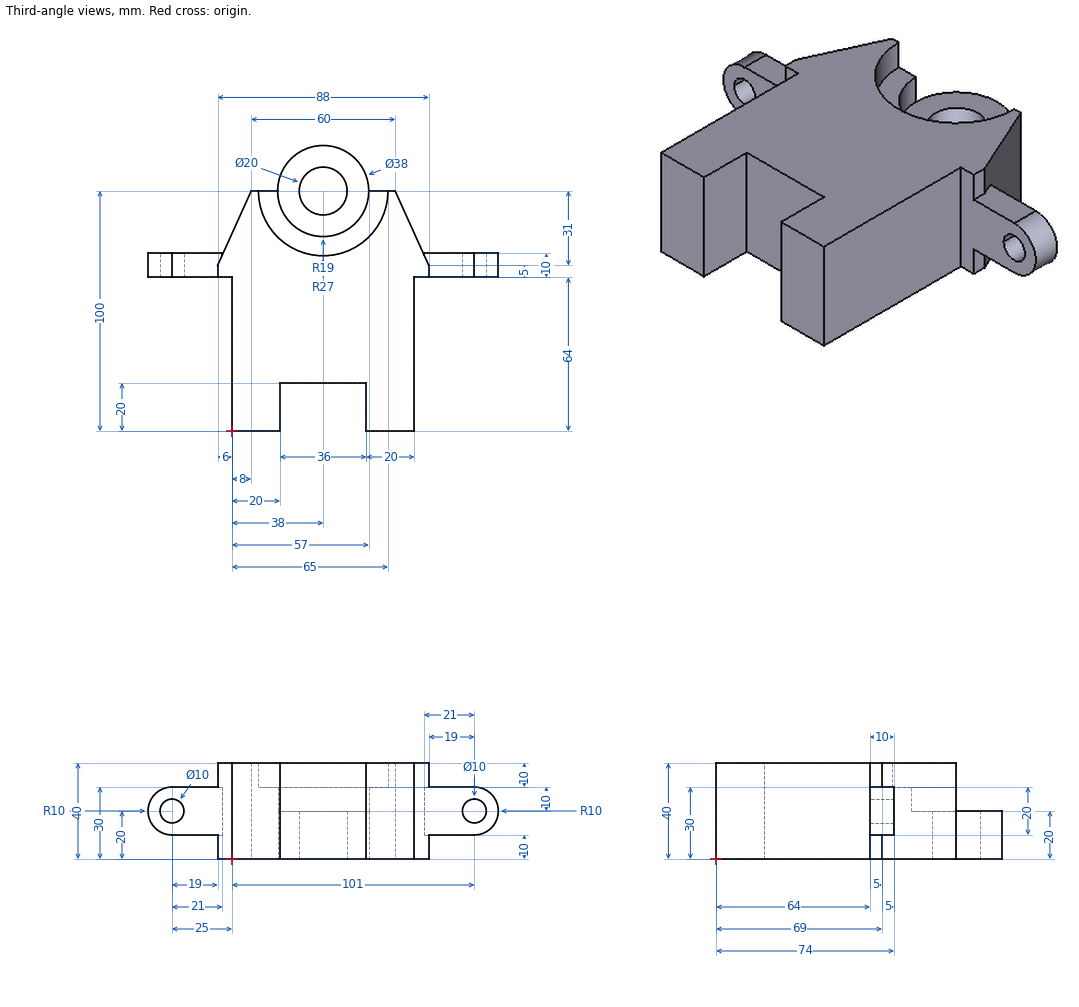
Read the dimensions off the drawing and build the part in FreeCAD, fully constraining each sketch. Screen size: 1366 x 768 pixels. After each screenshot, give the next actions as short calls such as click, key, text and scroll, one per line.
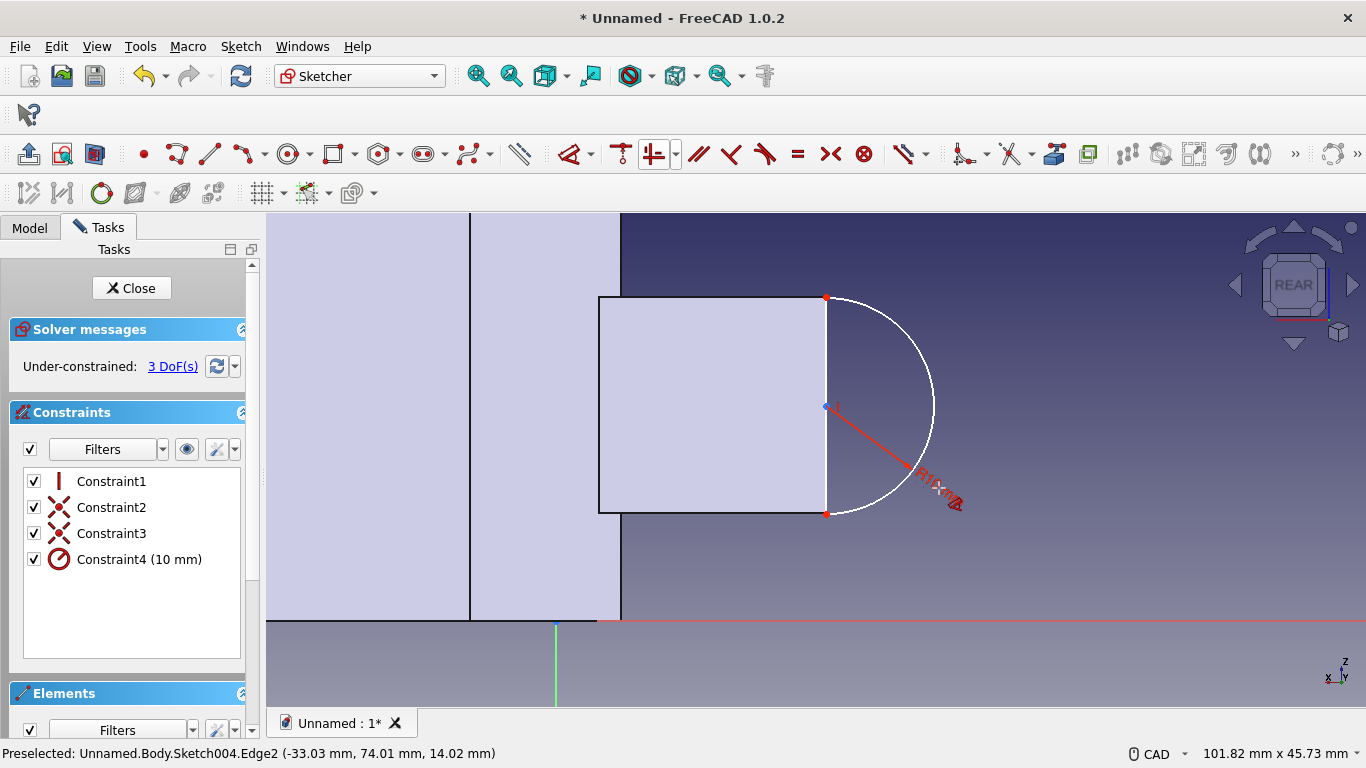
click(826, 298)
click(691, 655)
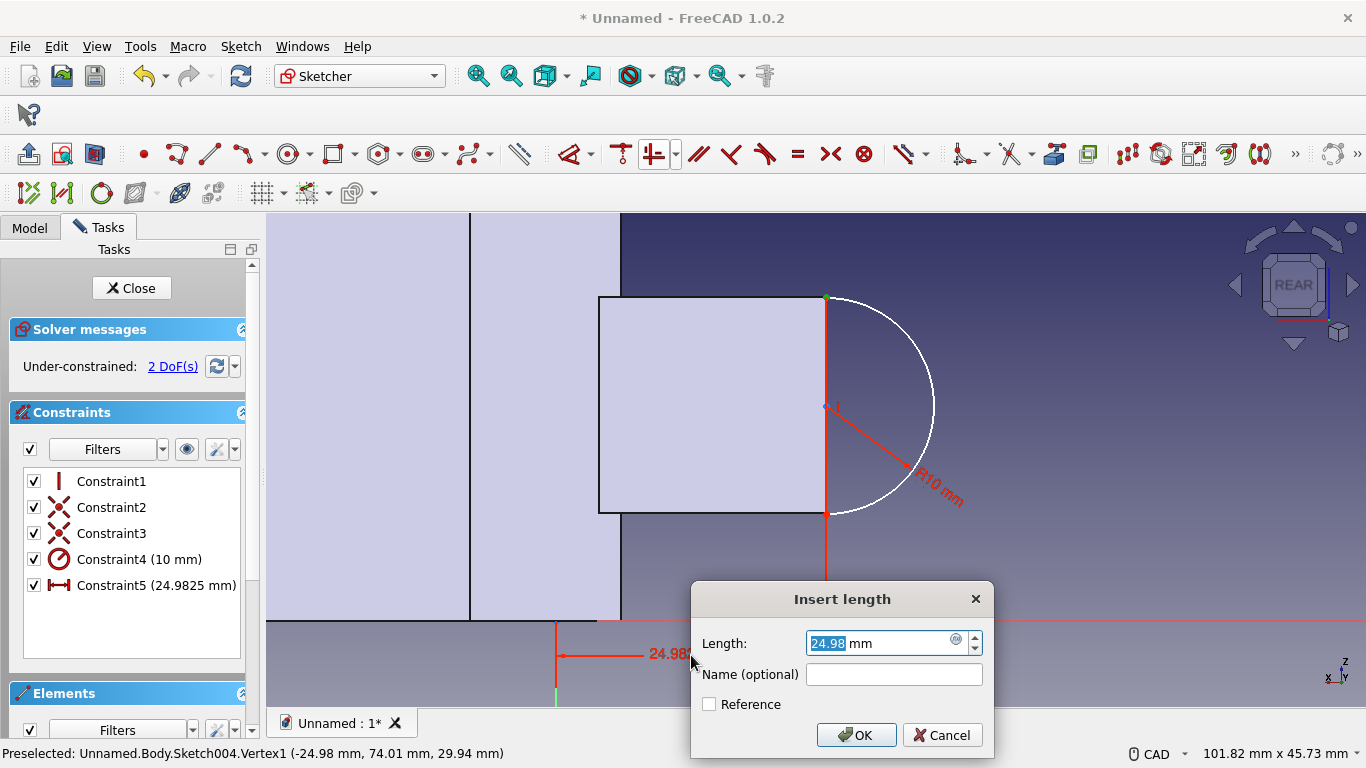
text(25)
key(Return)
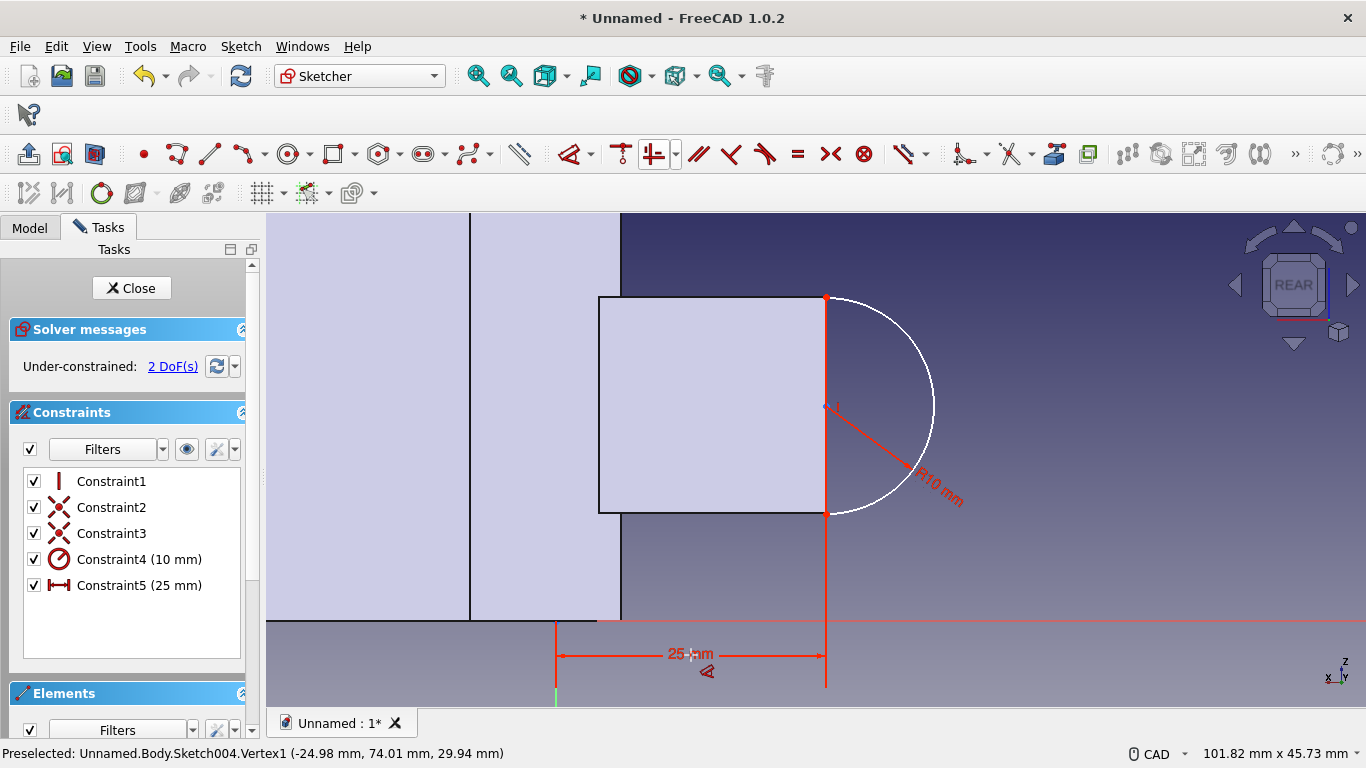
click(826, 298)
click(522, 460)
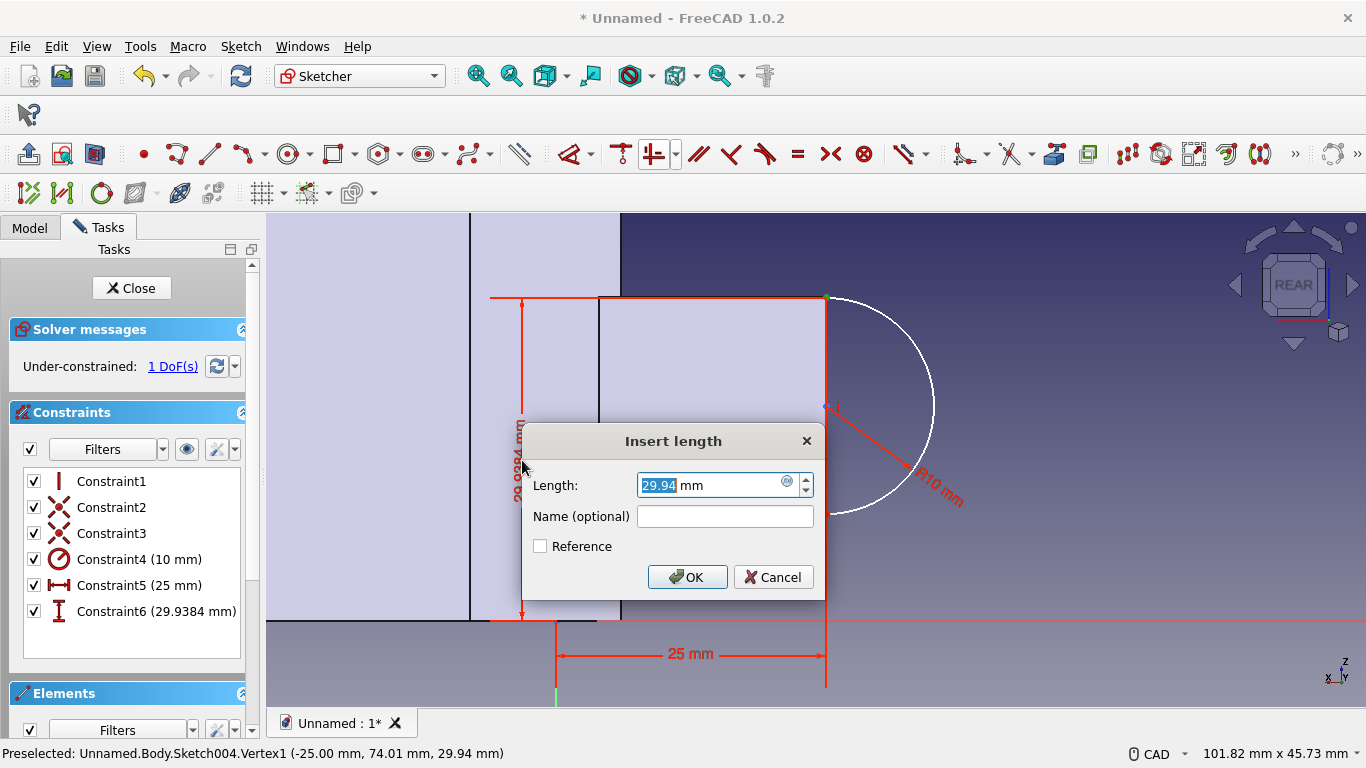
text(30)
key(Return)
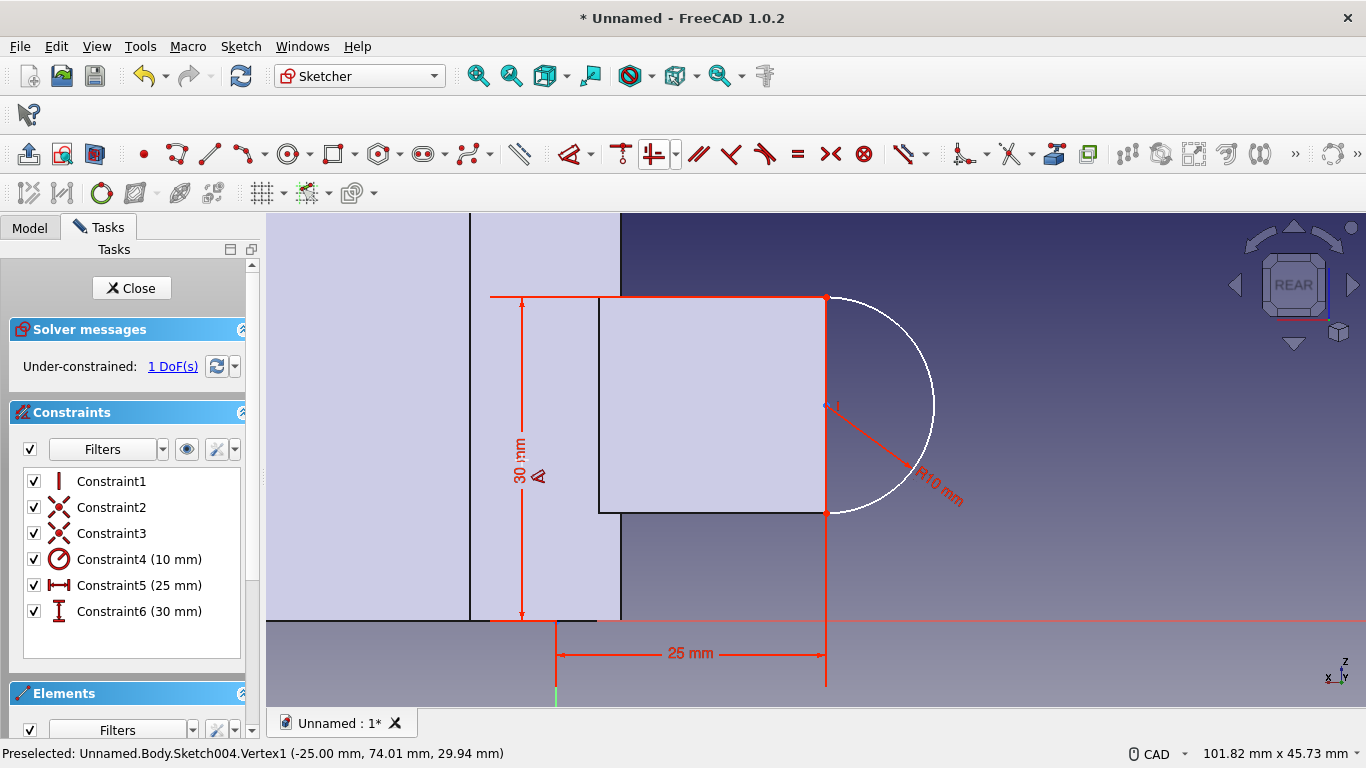
click(826, 405)
click(597, 655)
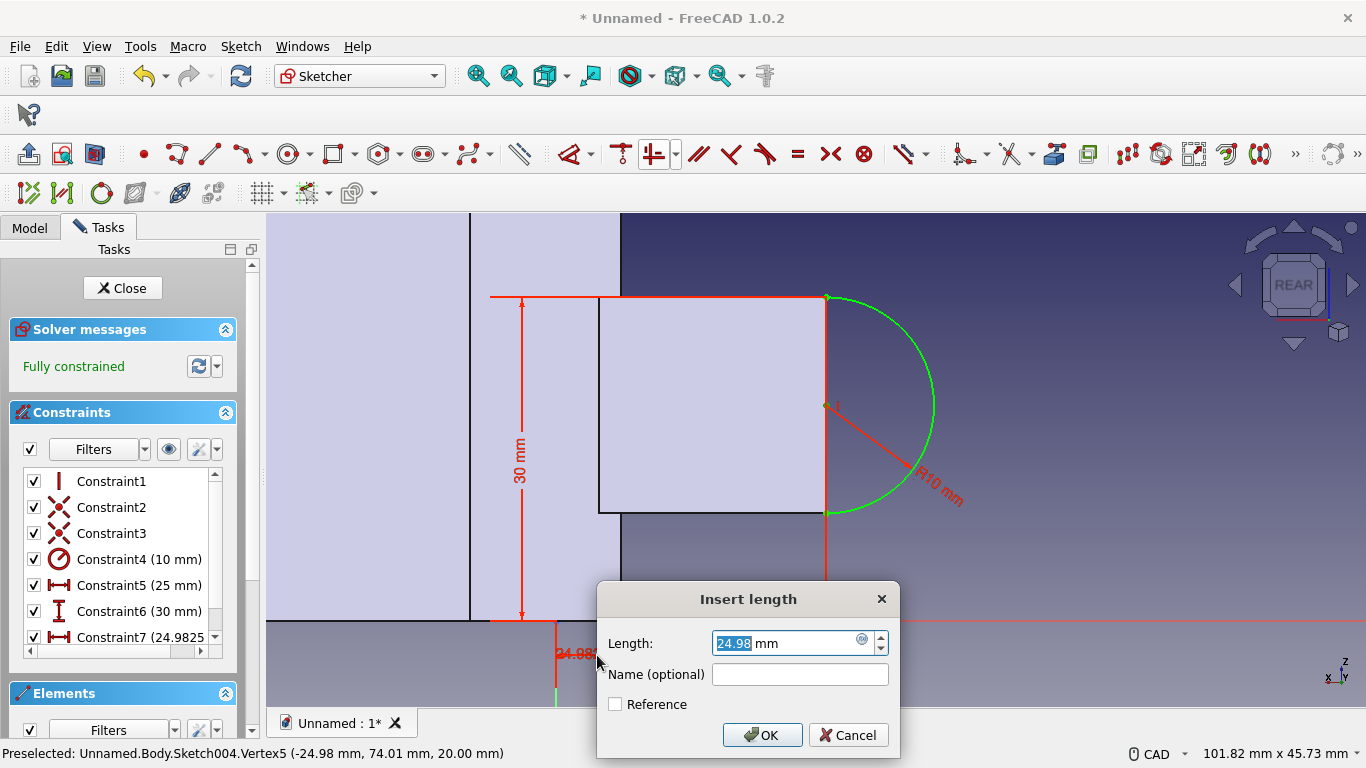
text(25)
key(Return)
key(Escape)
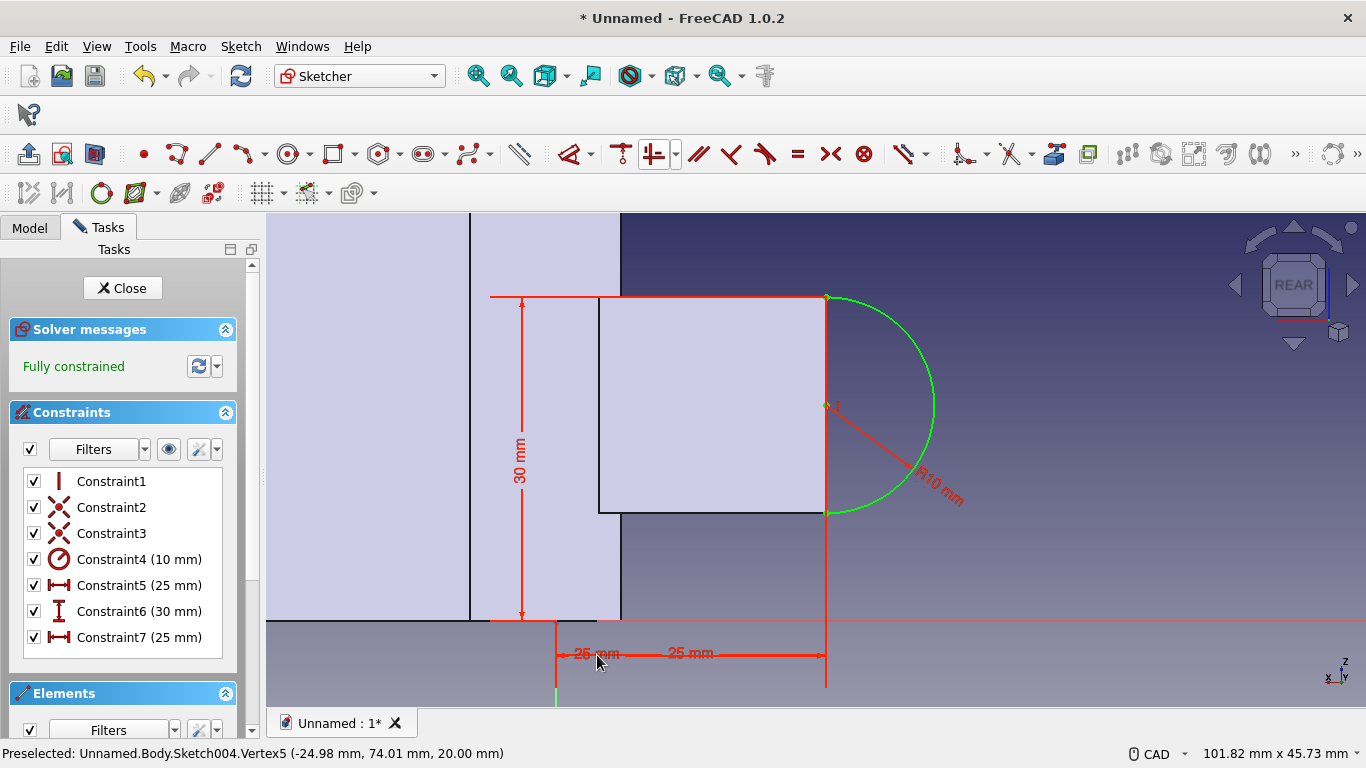
click(123, 288)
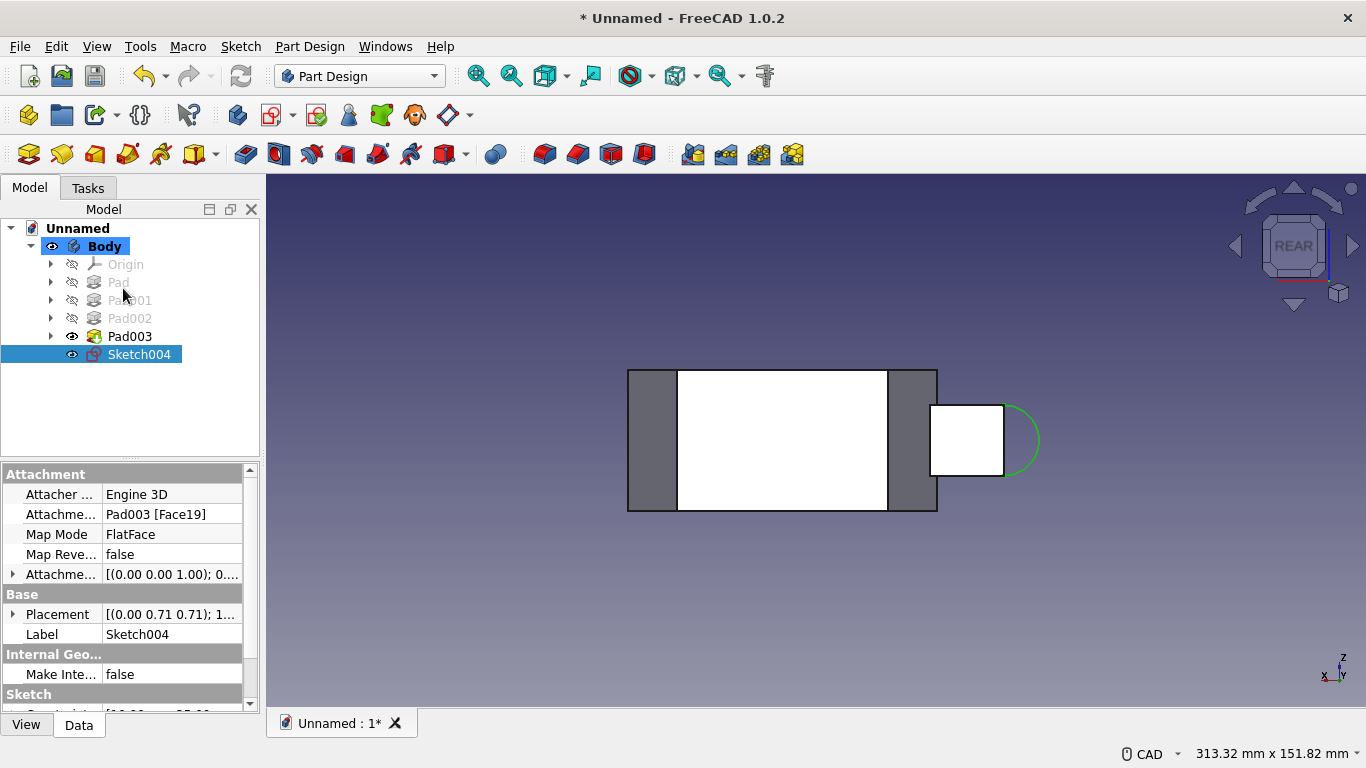
click(29, 154)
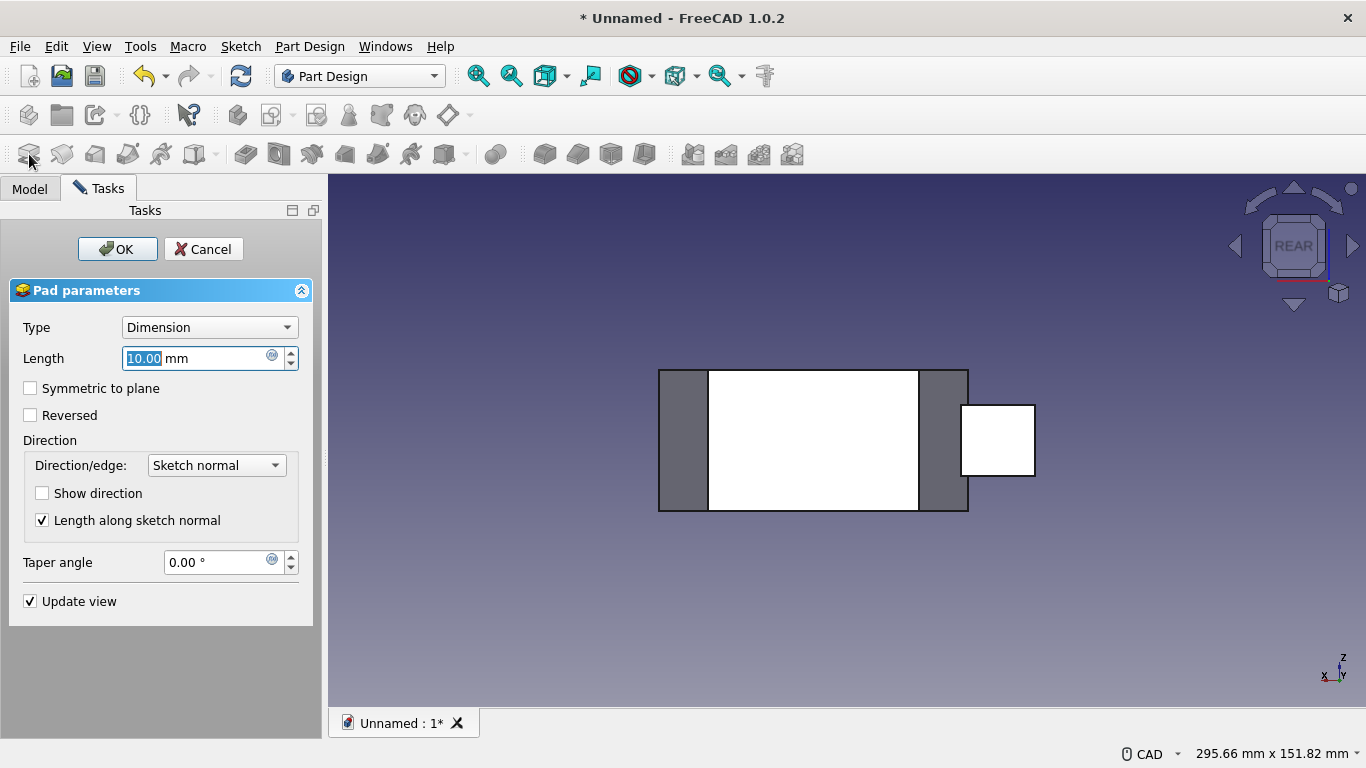
text(10)
key(Tab)